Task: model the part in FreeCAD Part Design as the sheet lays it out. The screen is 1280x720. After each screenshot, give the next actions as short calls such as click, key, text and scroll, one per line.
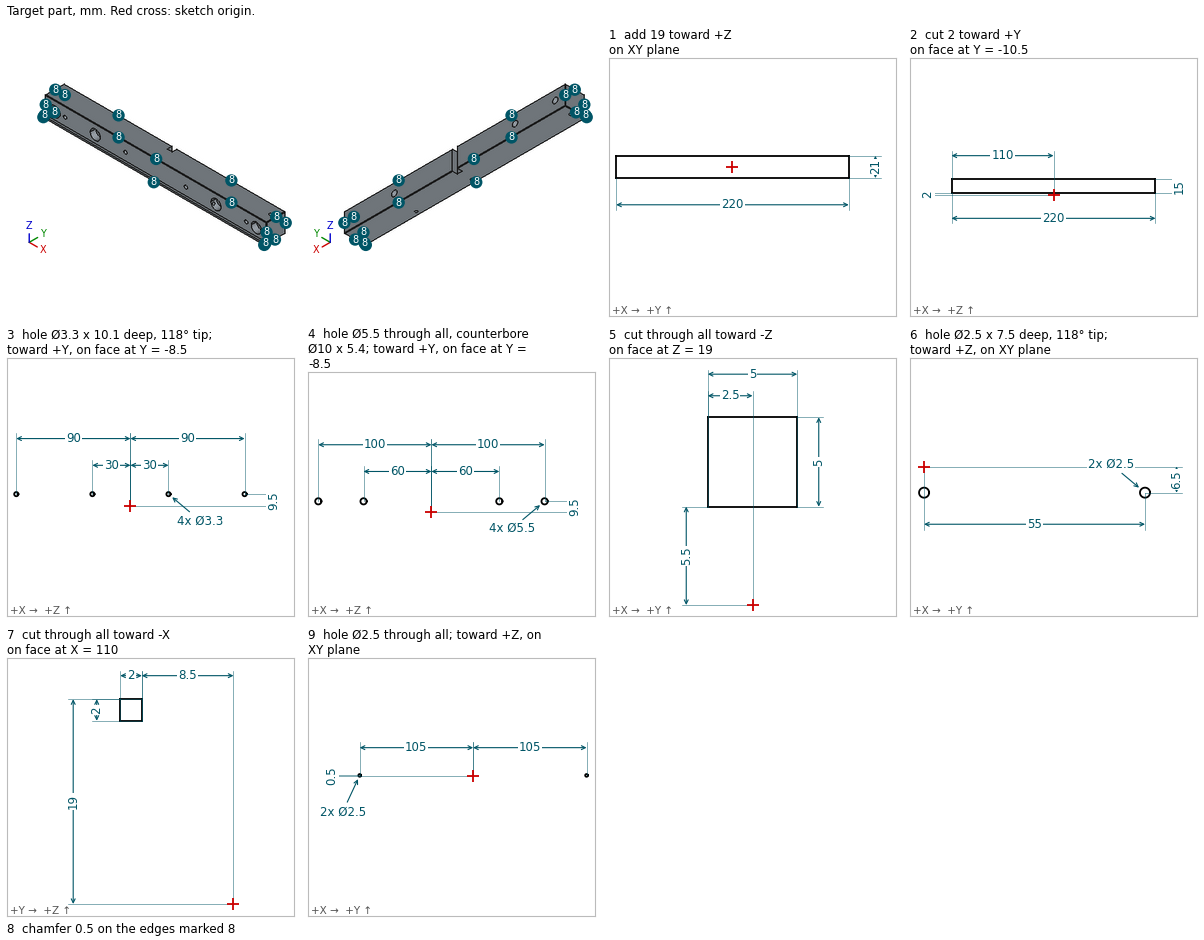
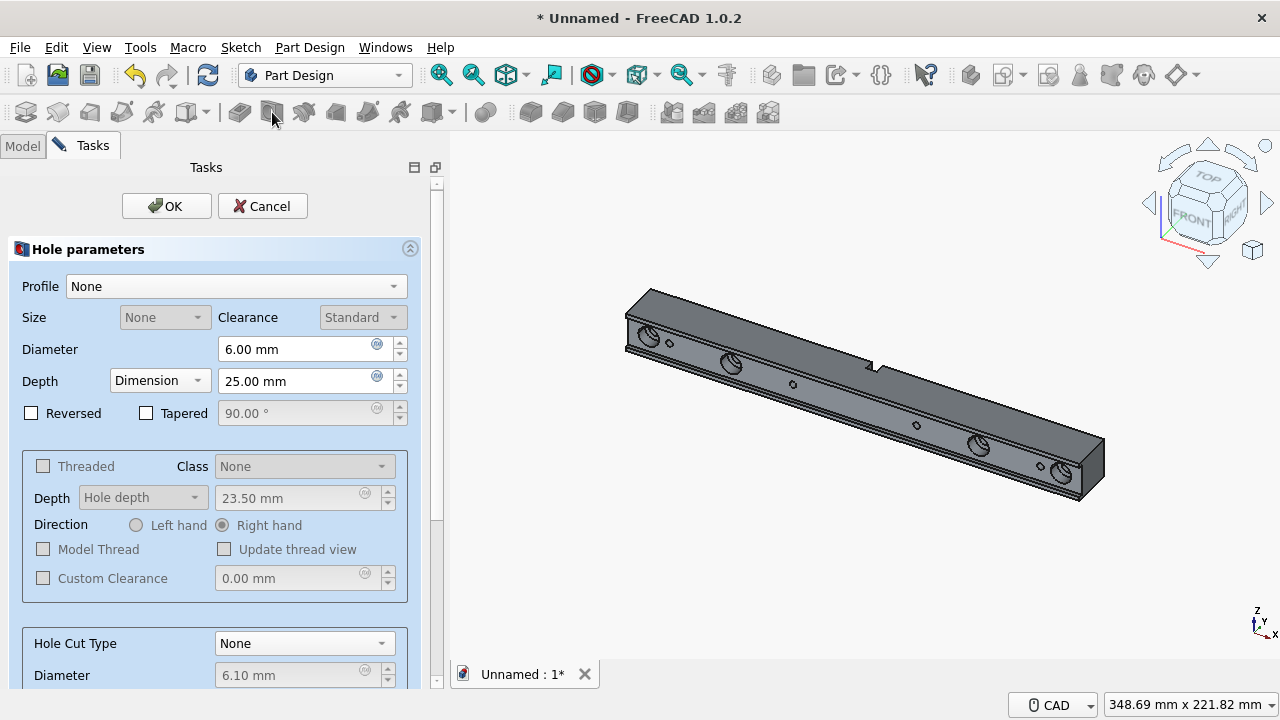
triple_click(305, 349)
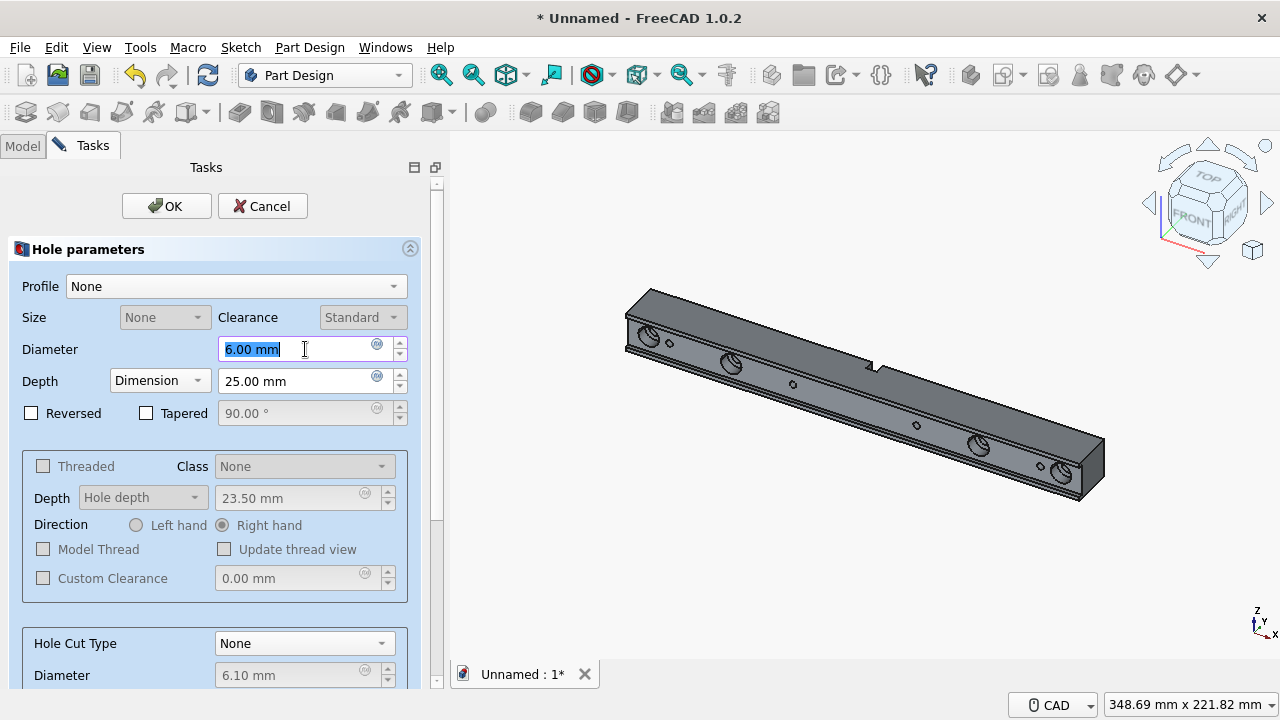
text(2.5)
key(Tab)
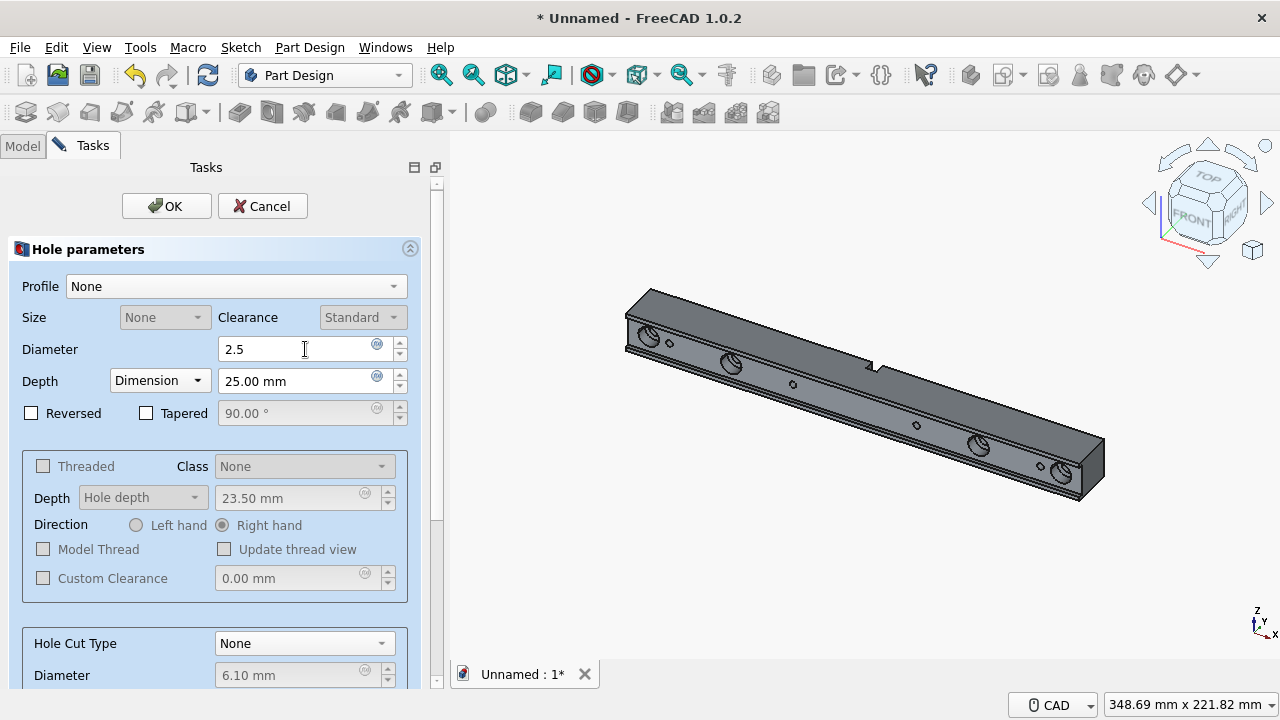
triple_click(305, 381)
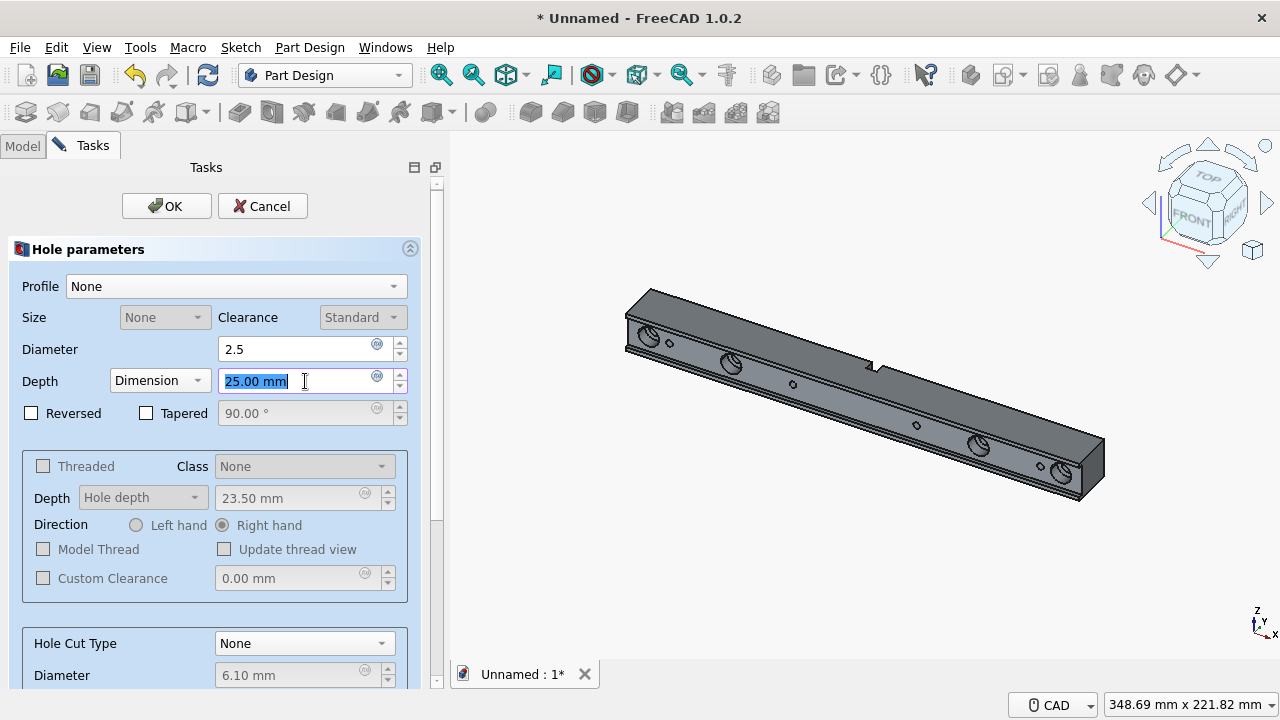
text(7.5)
key(Tab)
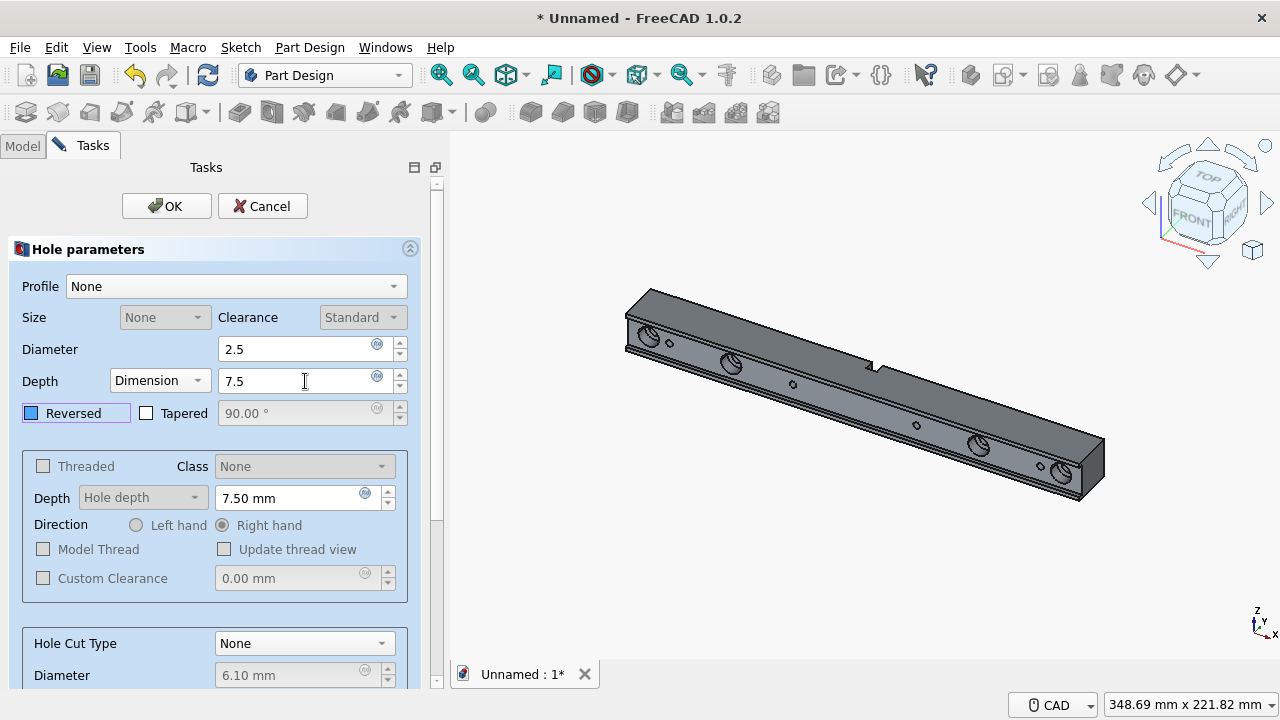
click(30, 413)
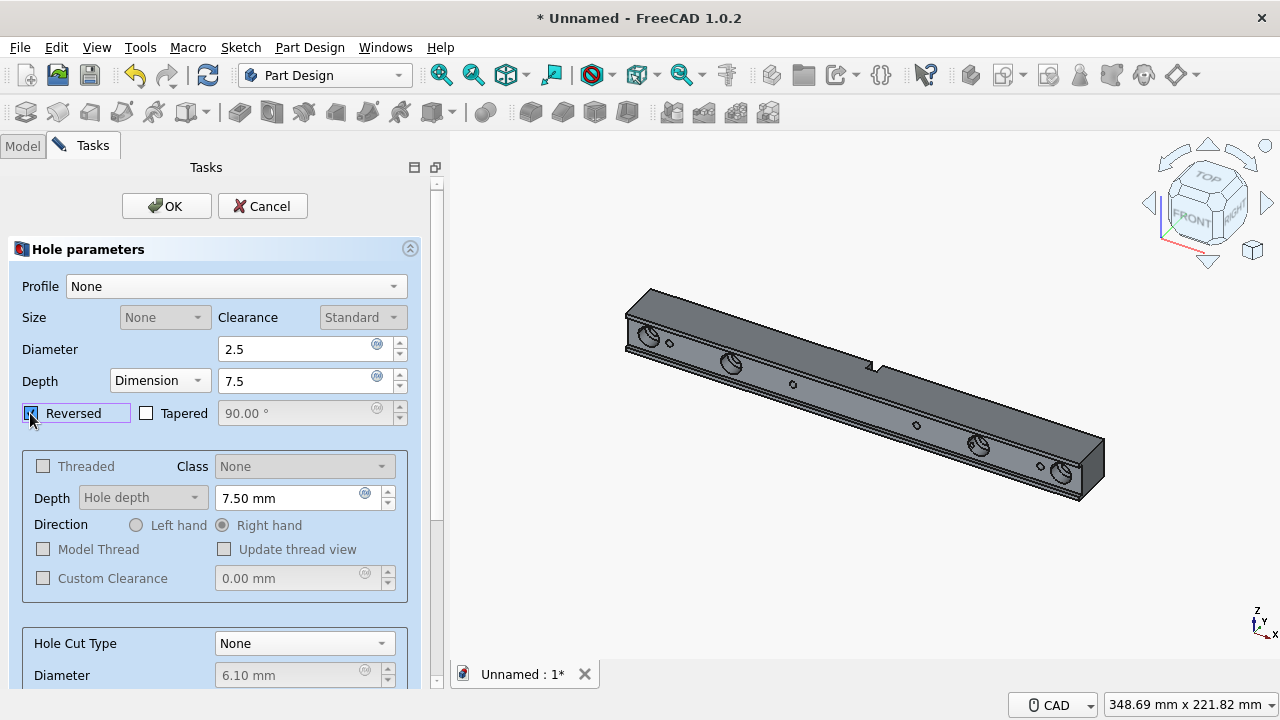
click(167, 206)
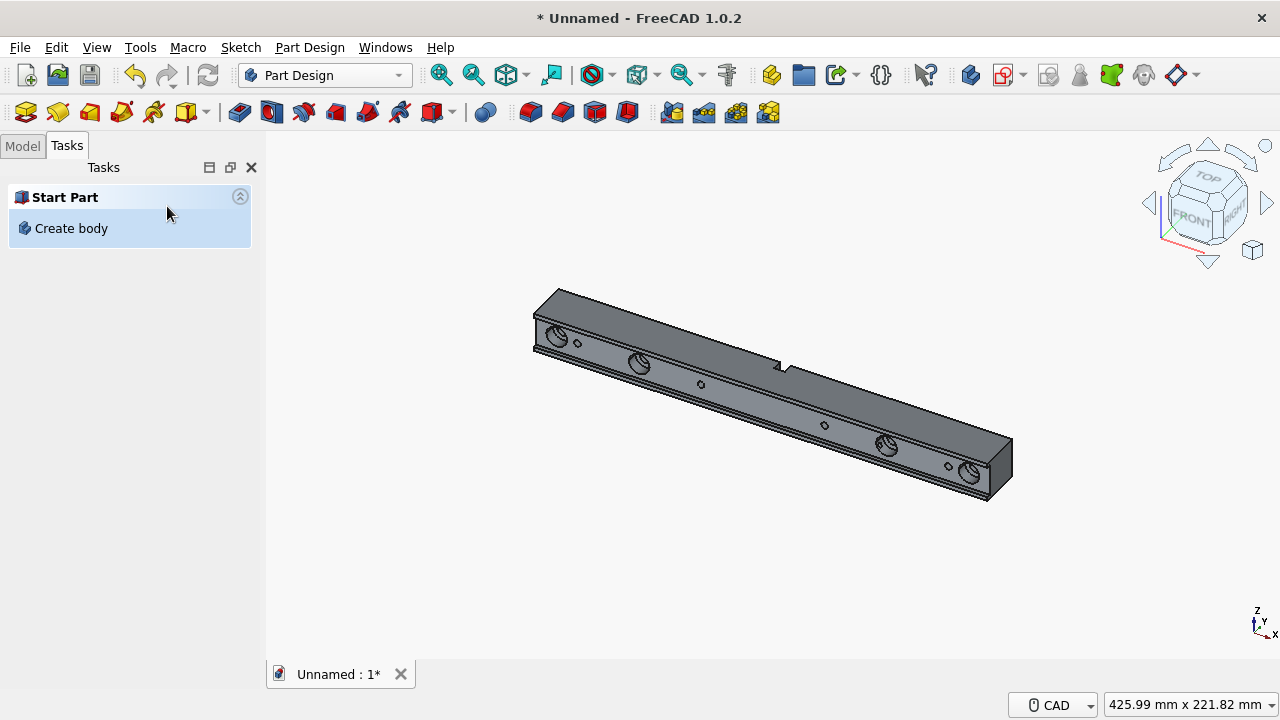
click(1000, 469)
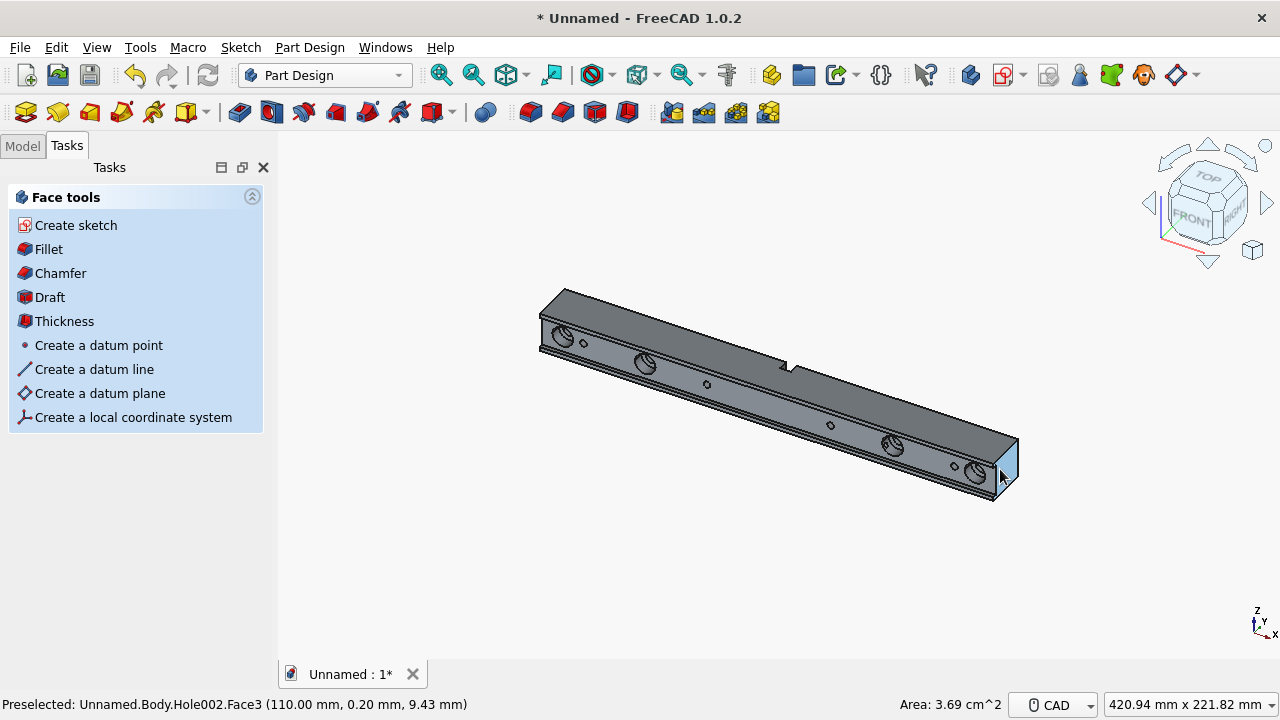
click(1004, 76)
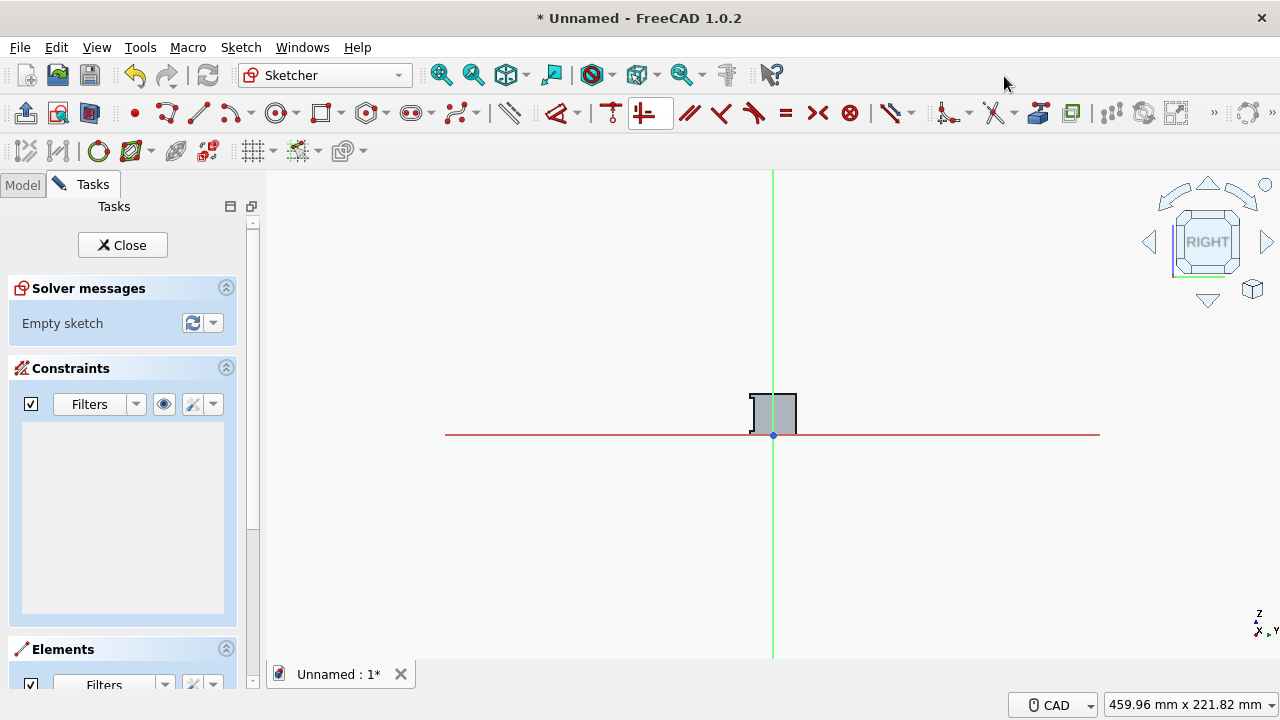
scroll(755, 395, up, 15)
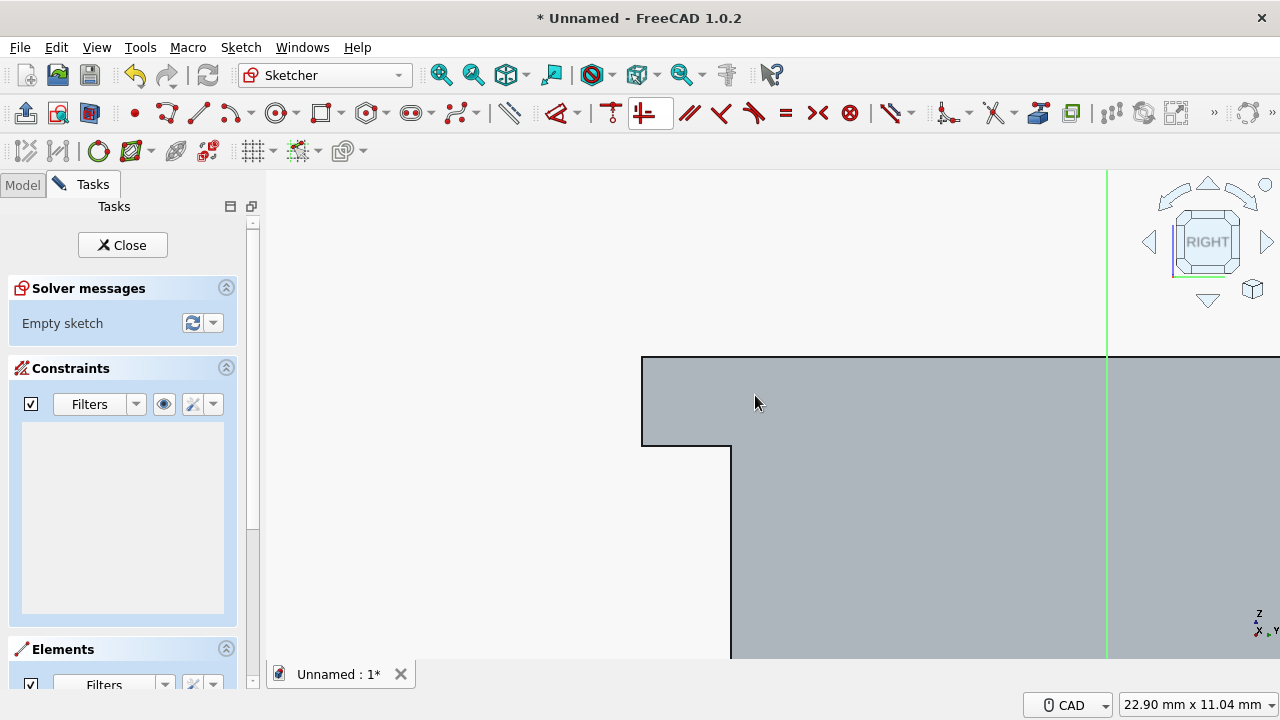
scroll(679, 396, up, 6)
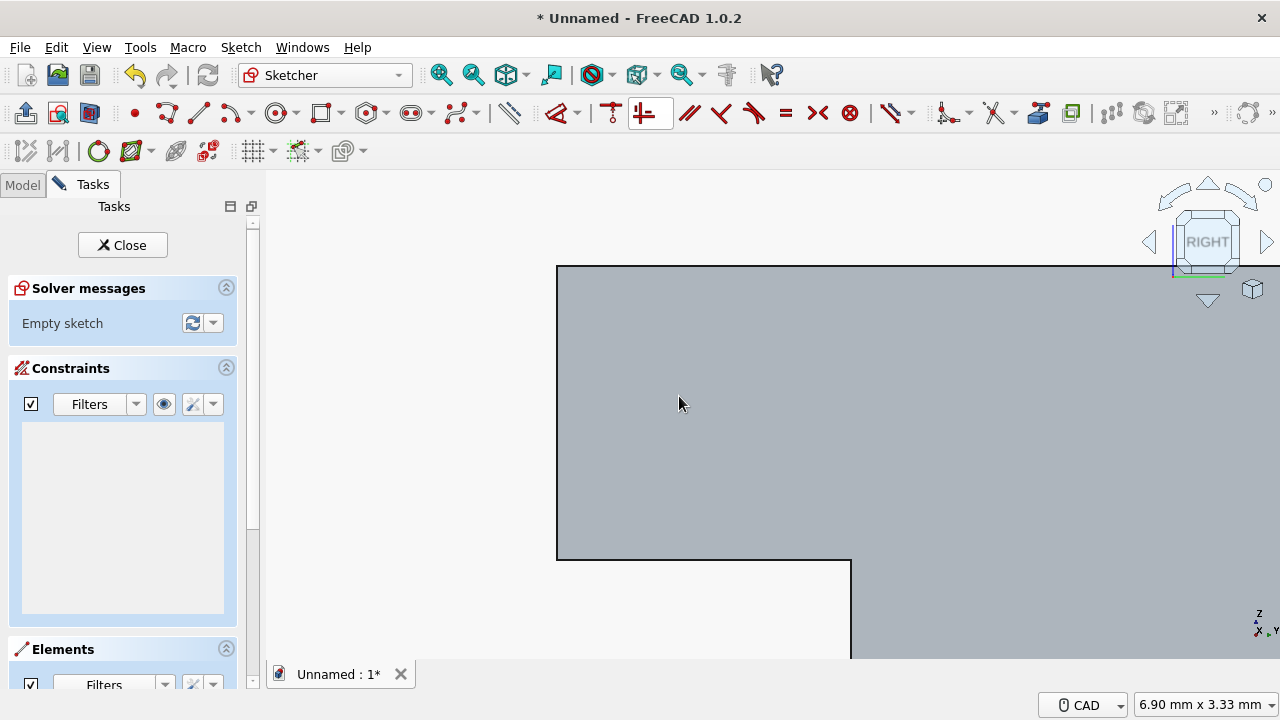
click(322, 114)